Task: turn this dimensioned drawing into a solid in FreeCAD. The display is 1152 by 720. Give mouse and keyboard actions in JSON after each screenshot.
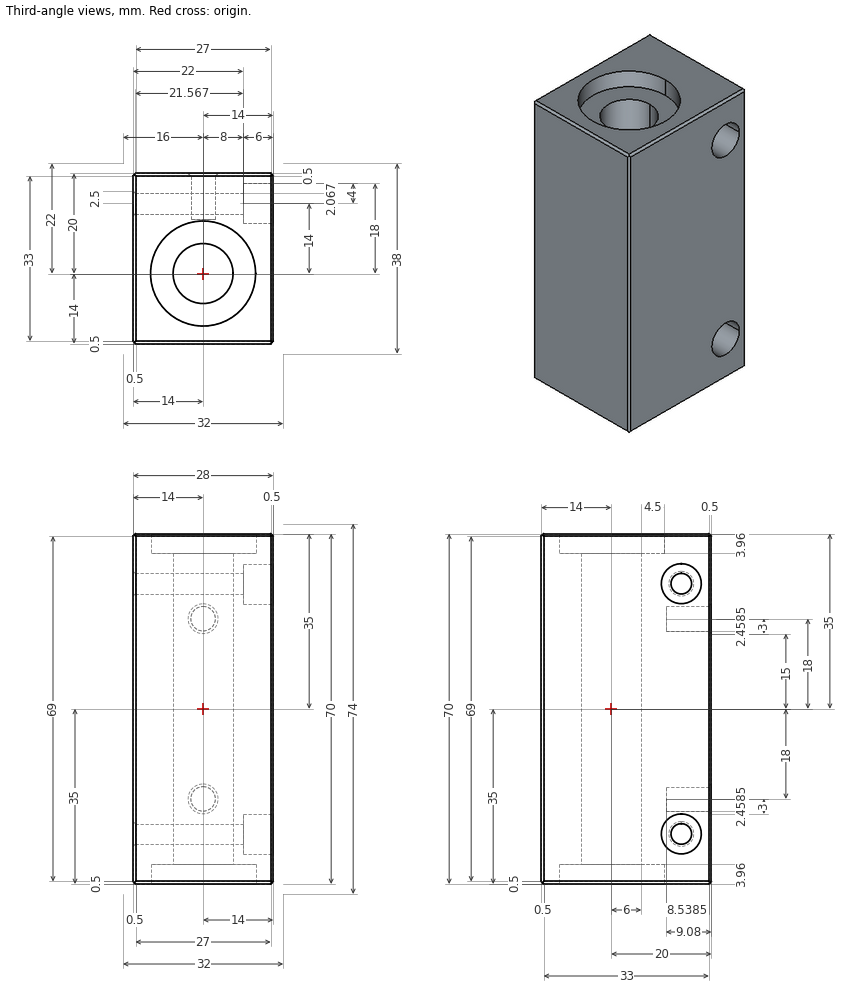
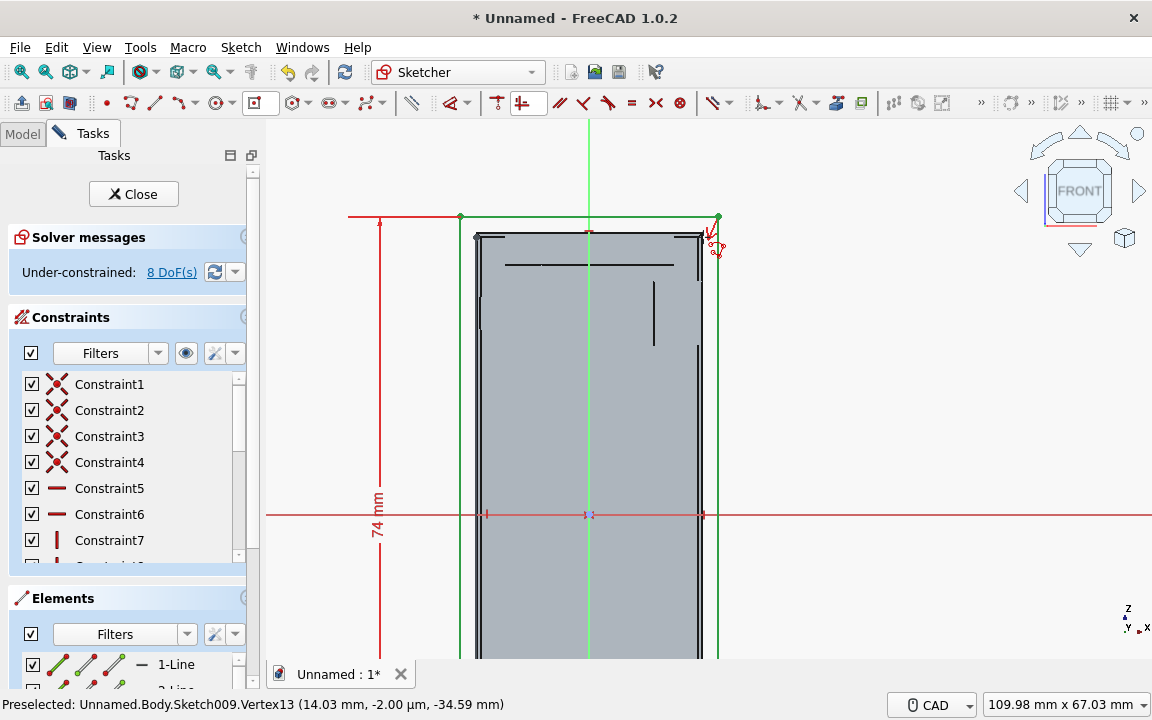
{"action": "left_click", "coordinate": [702, 237]}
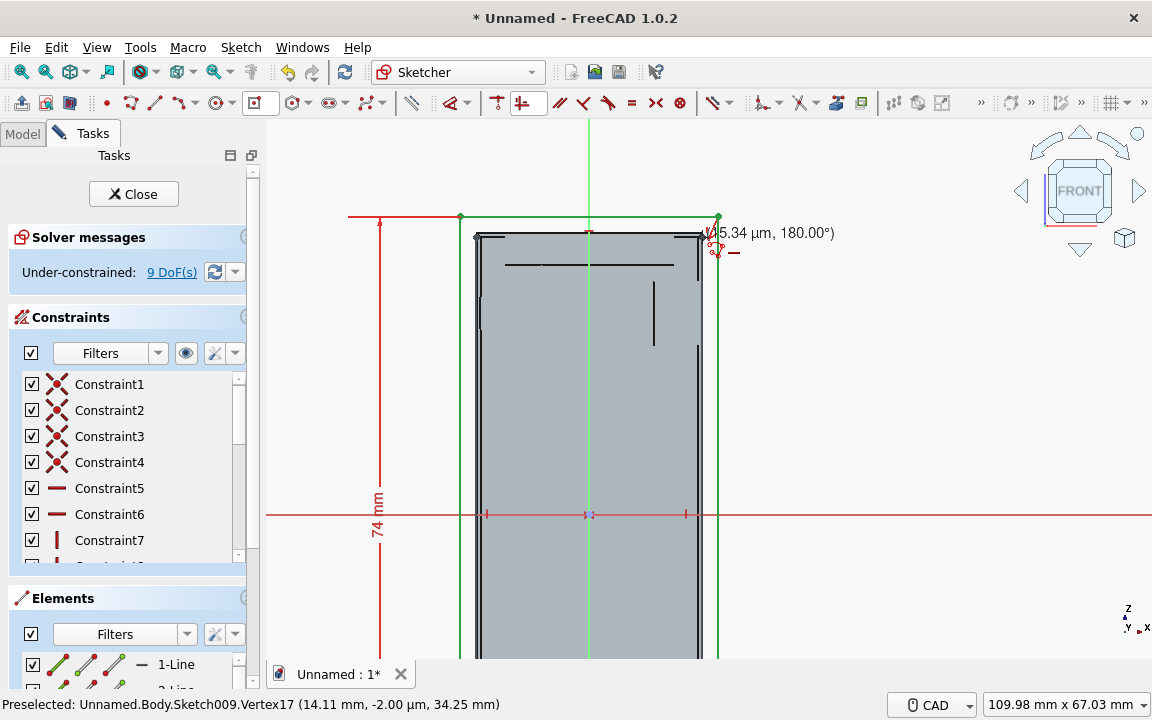
{"action": "scroll", "coordinate": [698, 233], "scroll_direction": "up", "scroll_amount": 6}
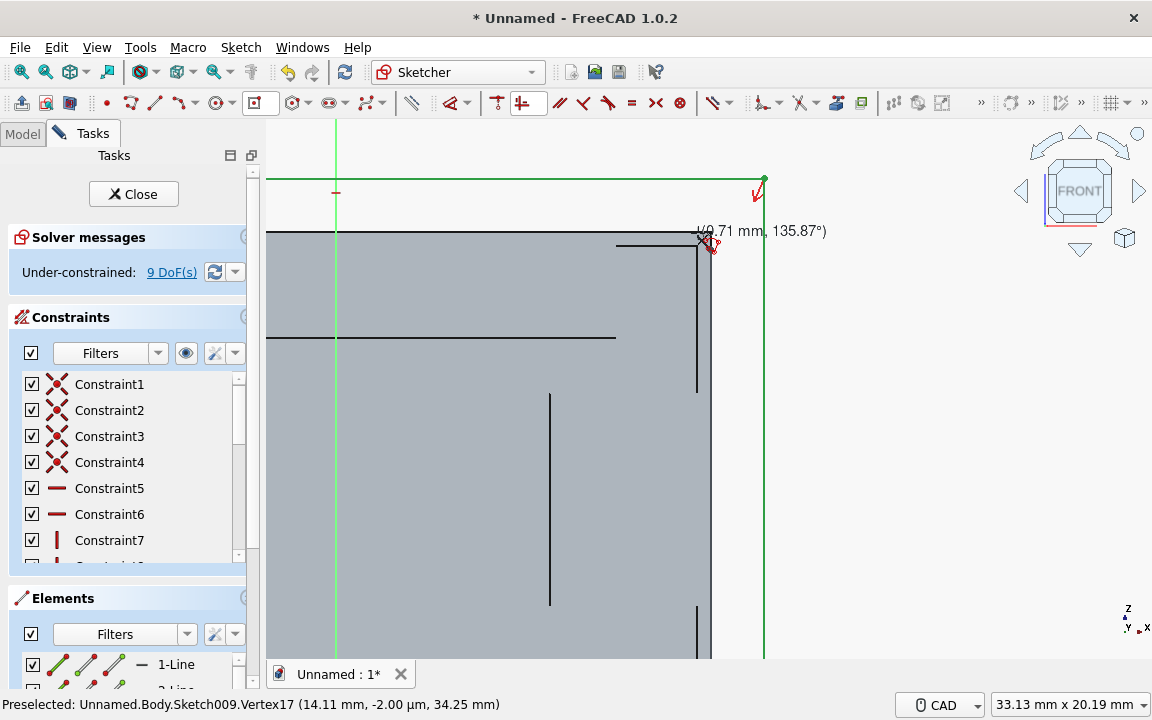
{"action": "left_click", "coordinate": [697, 232]}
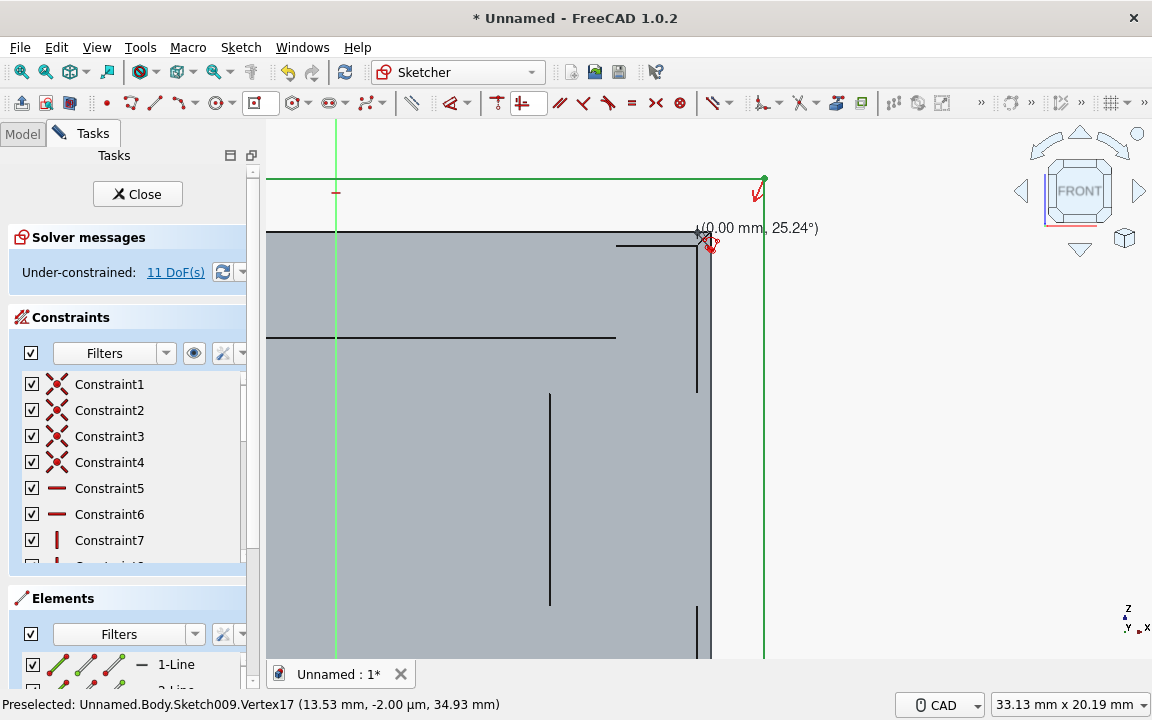
{"action": "scroll", "coordinate": [701, 235], "scroll_direction": "down", "scroll_amount": 9}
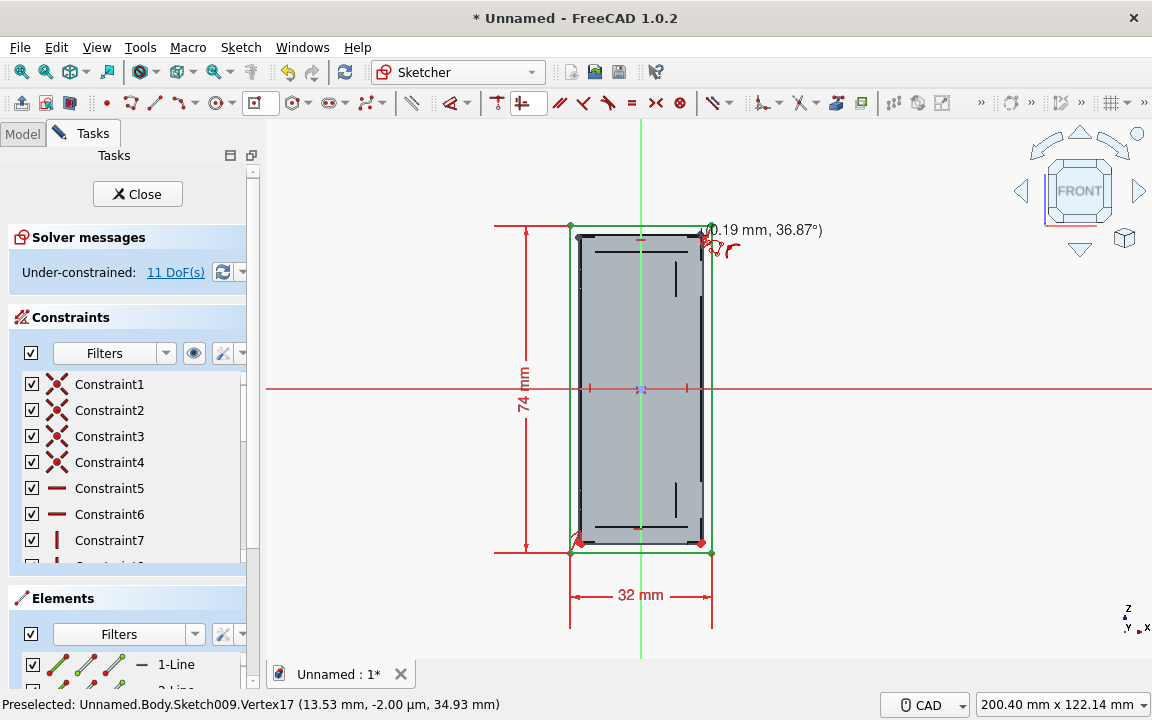
{"action": "scroll", "coordinate": [581, 235], "scroll_direction": "up", "scroll_amount": 9}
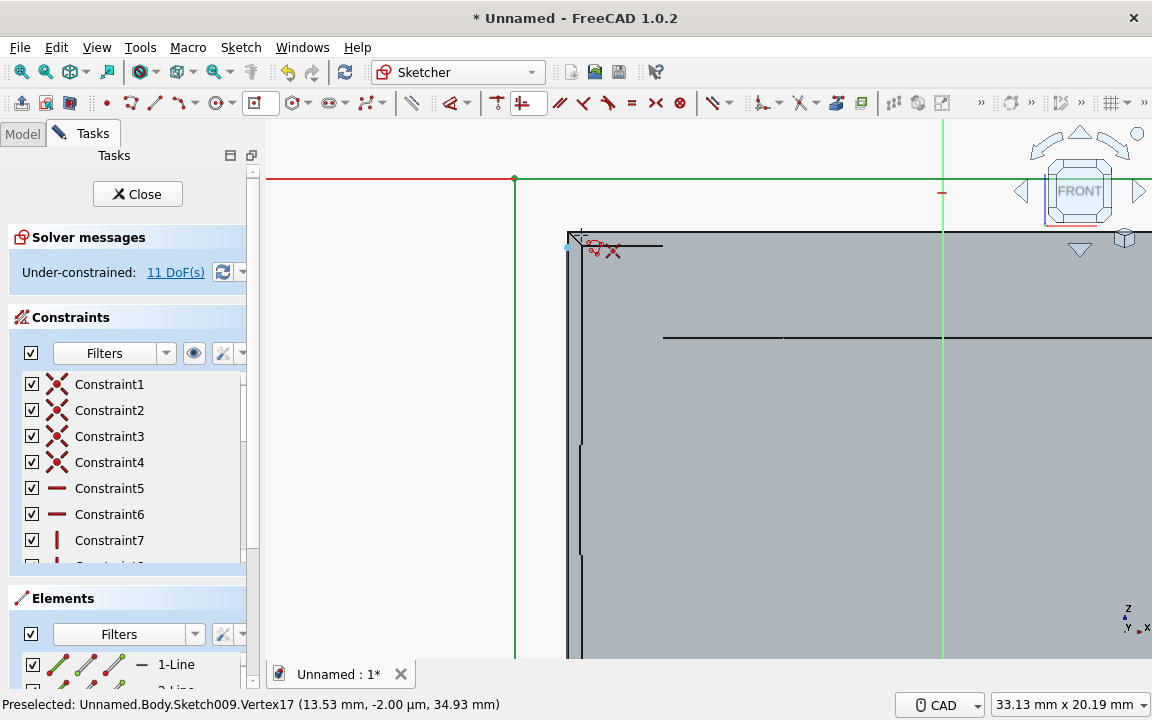
{"action": "left_click", "coordinate": [582, 232]}
{"action": "left_click", "coordinate": [567, 247]}
{"action": "key", "text": "Escape"}
{"action": "key", "text": "Escape"}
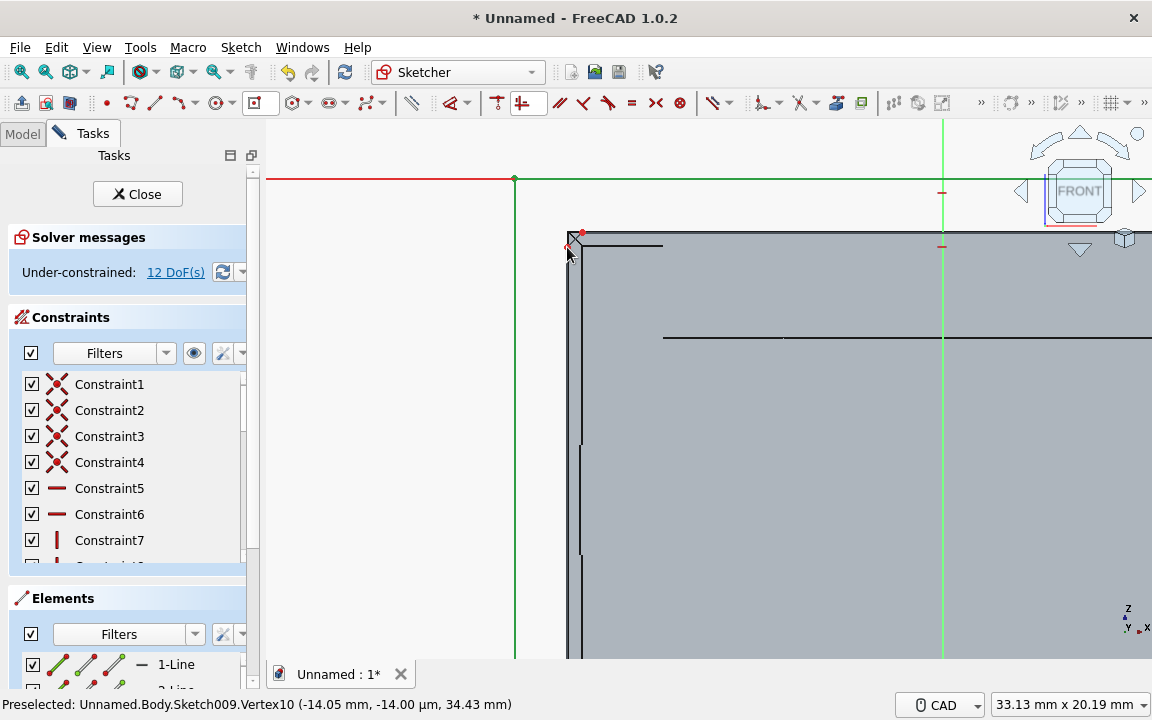
{"action": "left_click", "coordinate": [450, 104]}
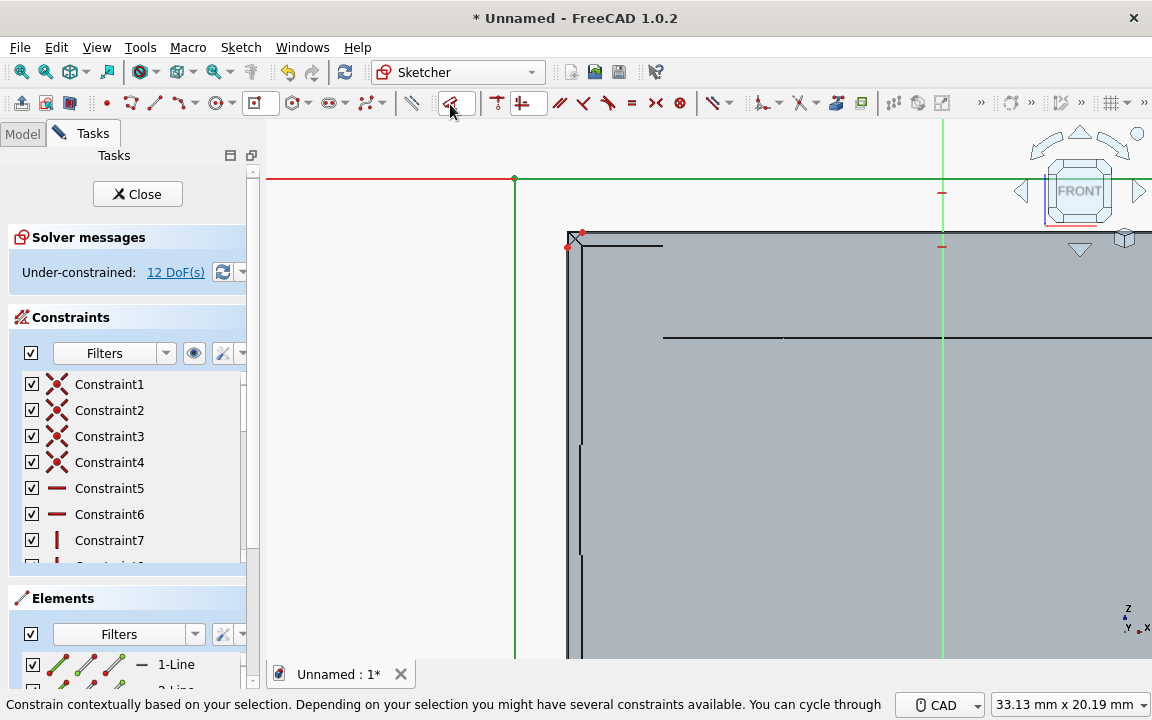
{"action": "scroll", "coordinate": [581, 235], "scroll_direction": "down", "scroll_amount": 9}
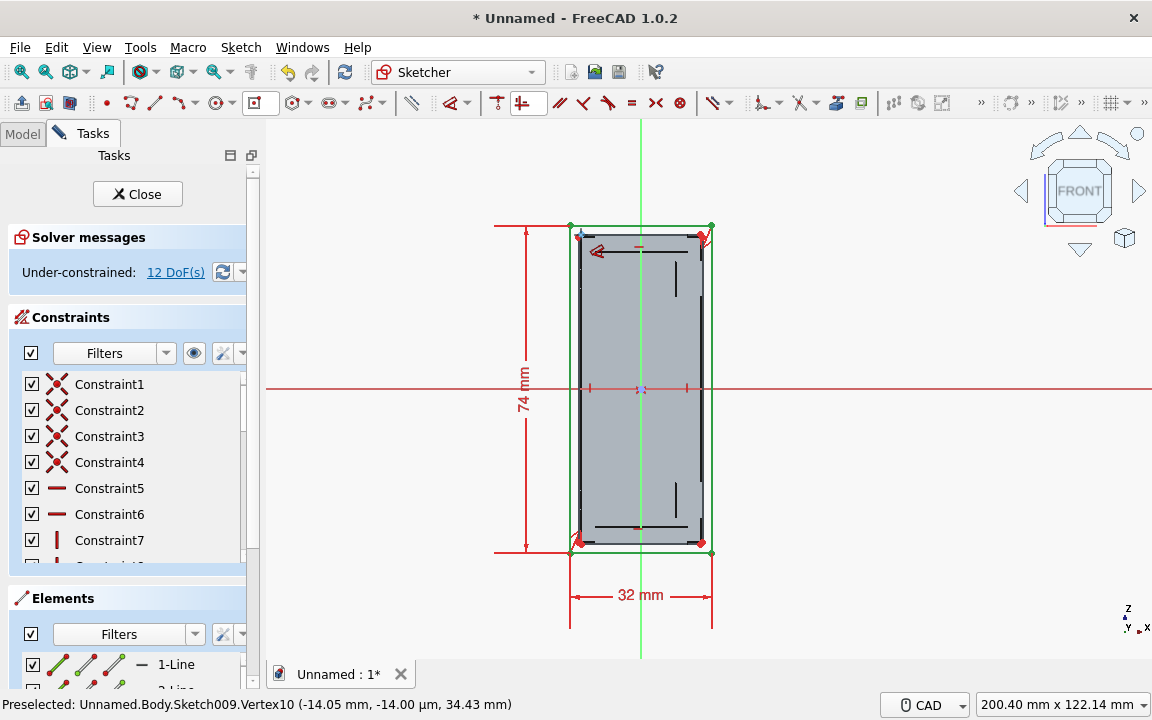
{"action": "scroll", "coordinate": [579, 298], "scroll_direction": "up", "scroll_amount": 3}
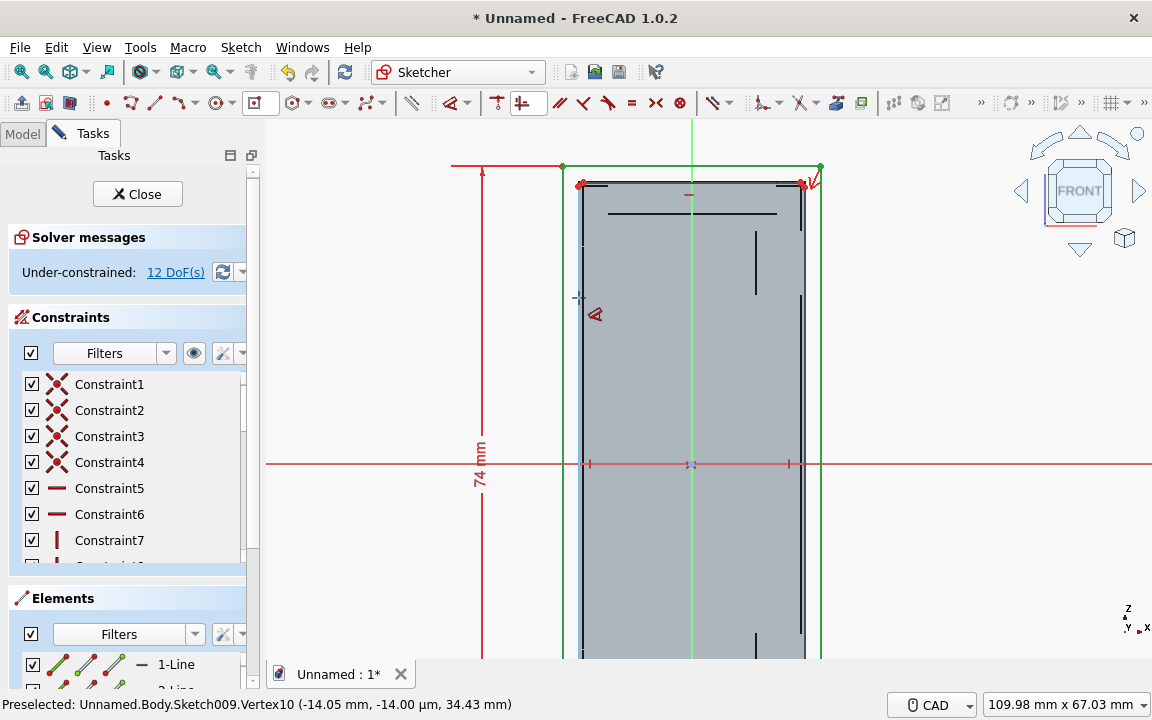
{"action": "left_click", "coordinate": [579, 298]}
{"action": "left_click", "coordinate": [545, 409]}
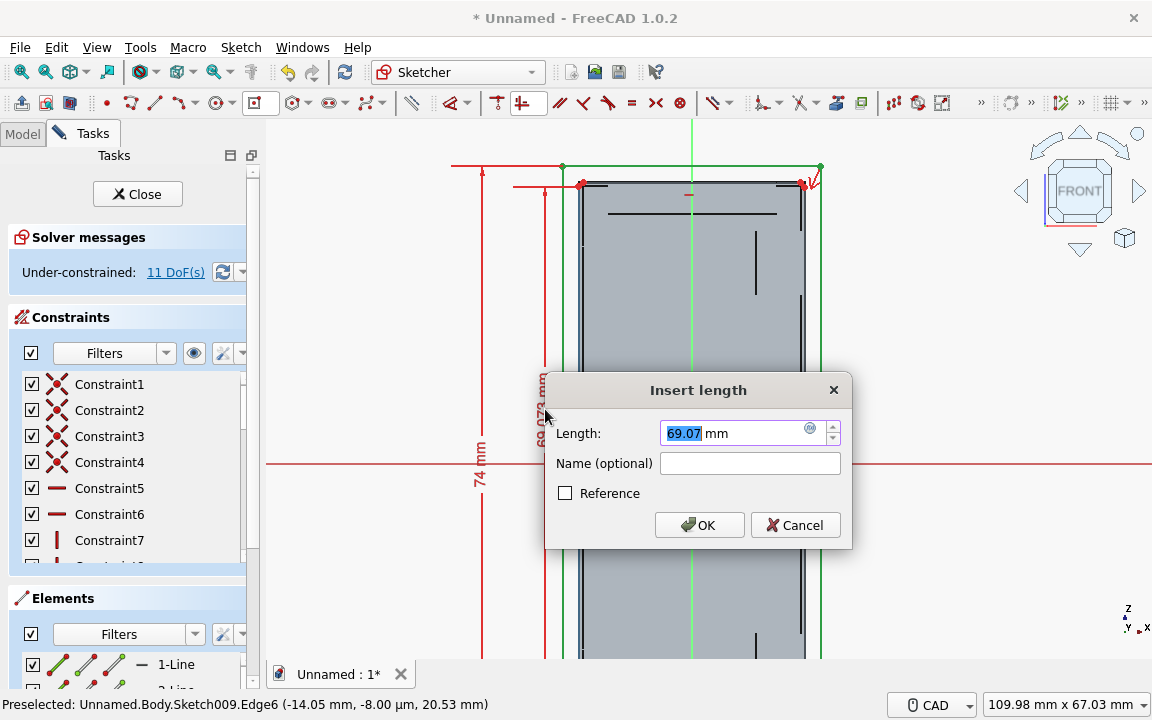
{"action": "type", "text": "69"}
{"action": "key", "text": "Return"}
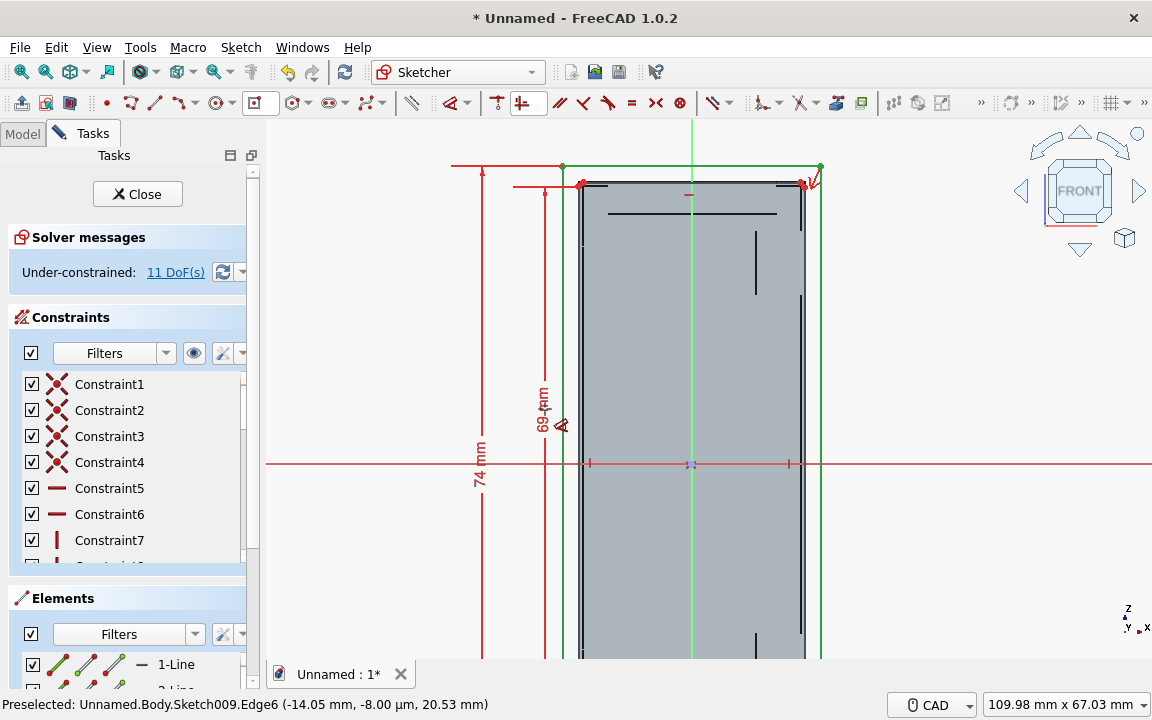
{"action": "scroll", "coordinate": [578, 297], "scroll_direction": "down", "scroll_amount": 3}